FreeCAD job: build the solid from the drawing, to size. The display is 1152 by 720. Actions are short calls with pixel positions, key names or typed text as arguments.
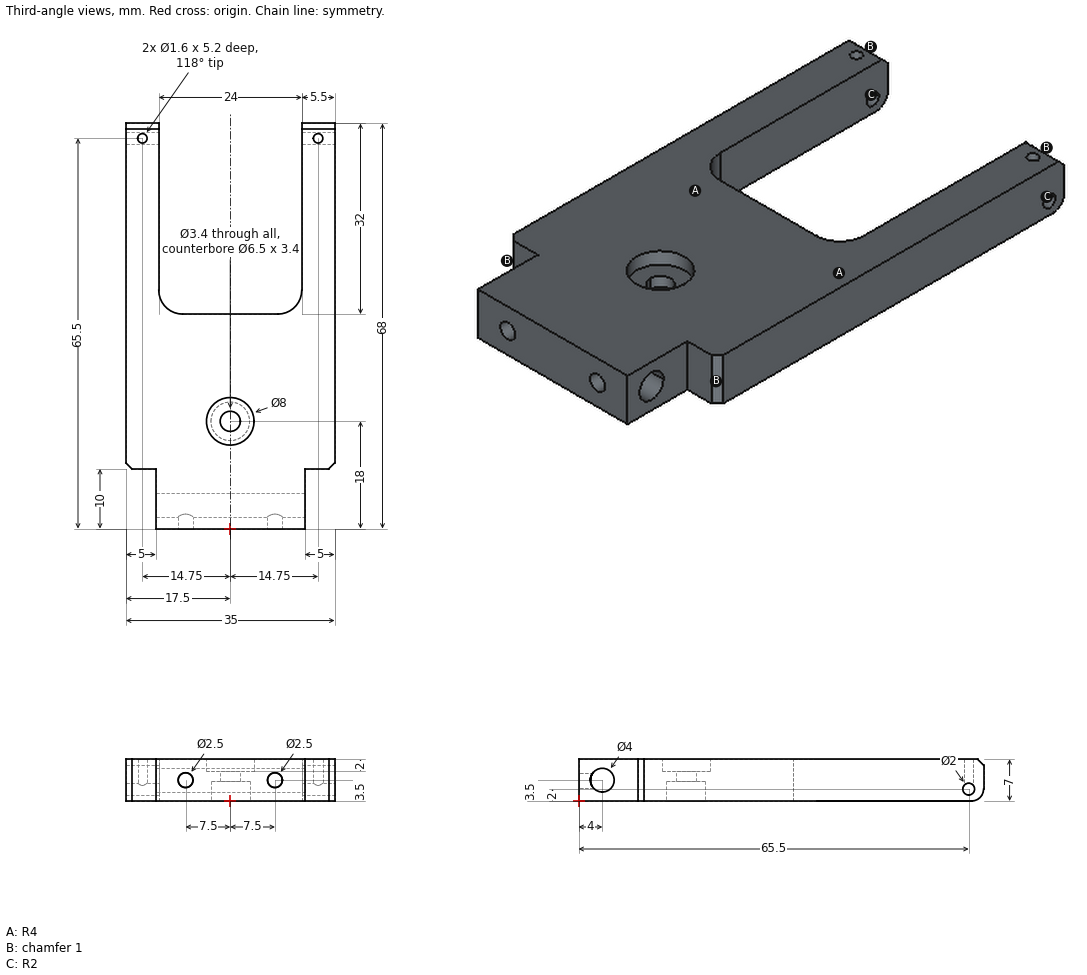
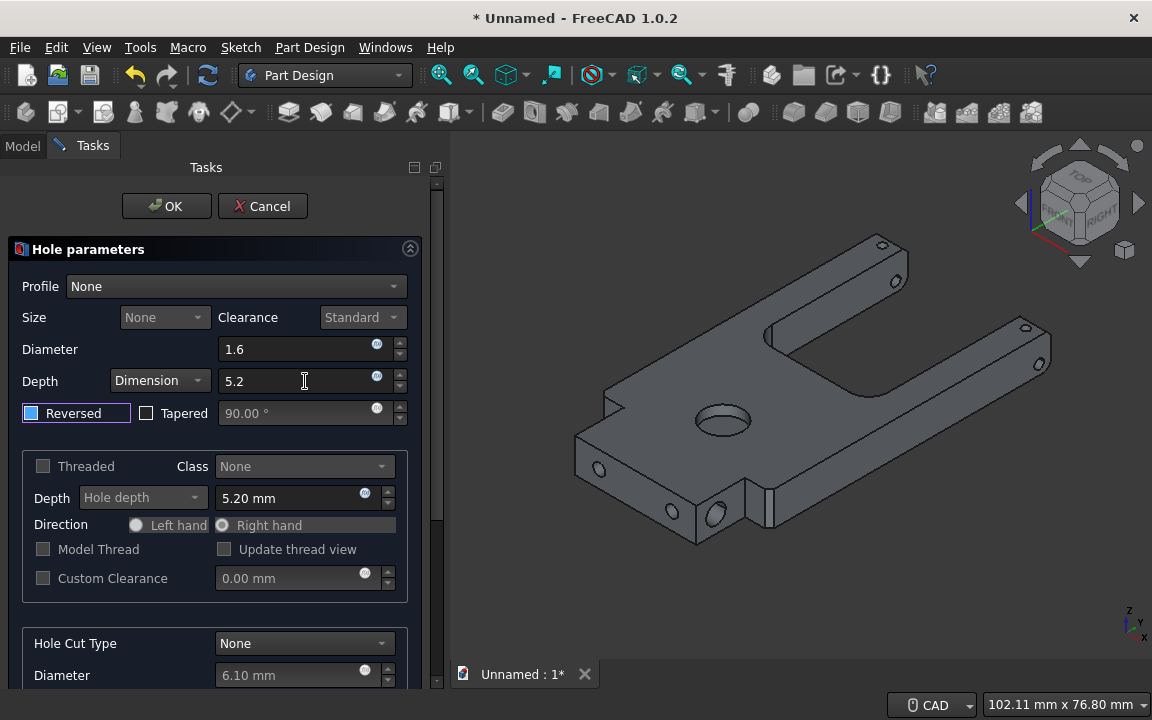
click(167, 206)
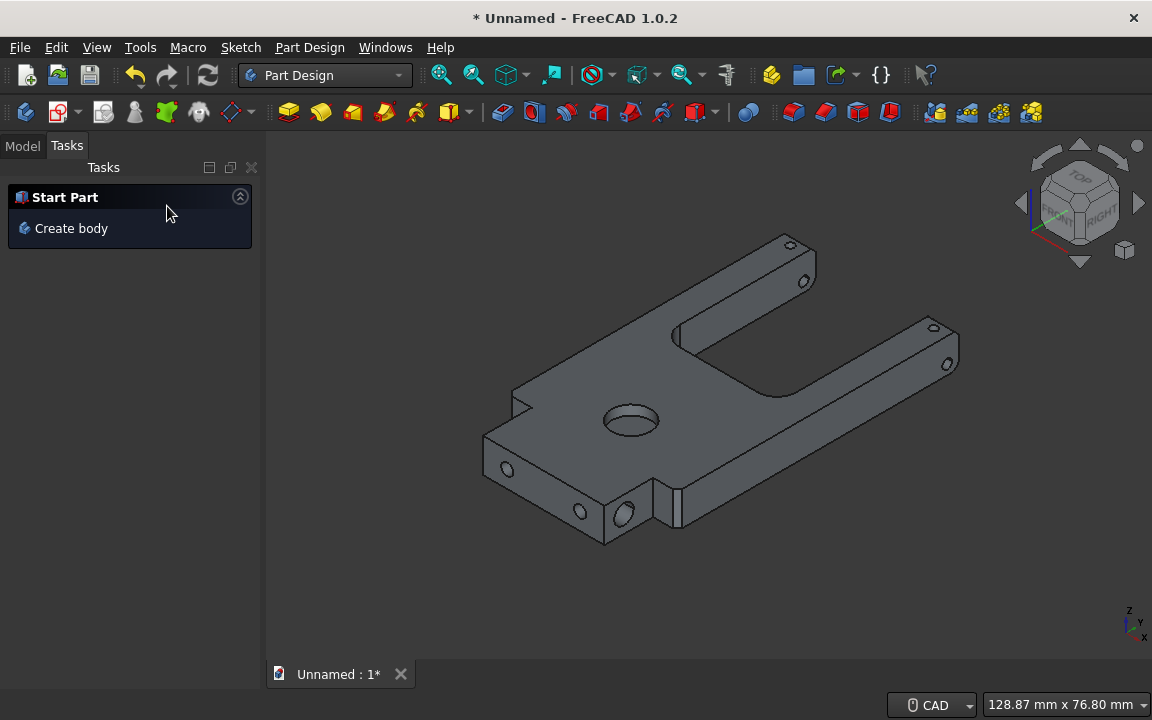
key(5)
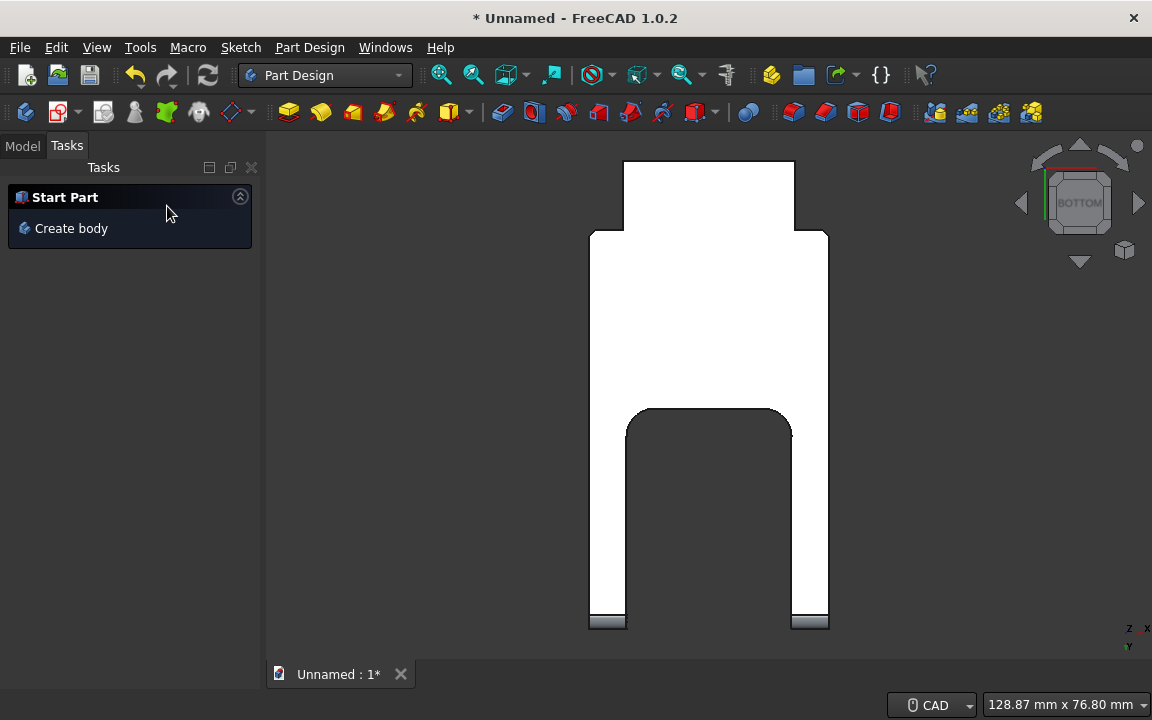
click(709, 257)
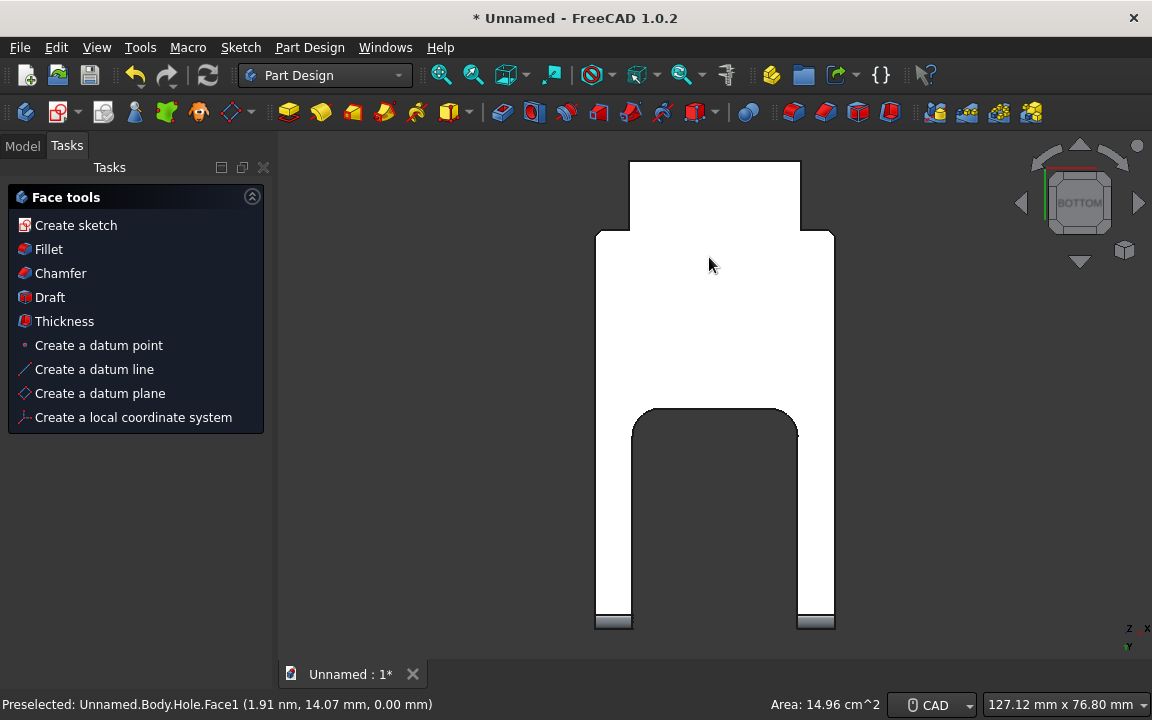
click(58, 112)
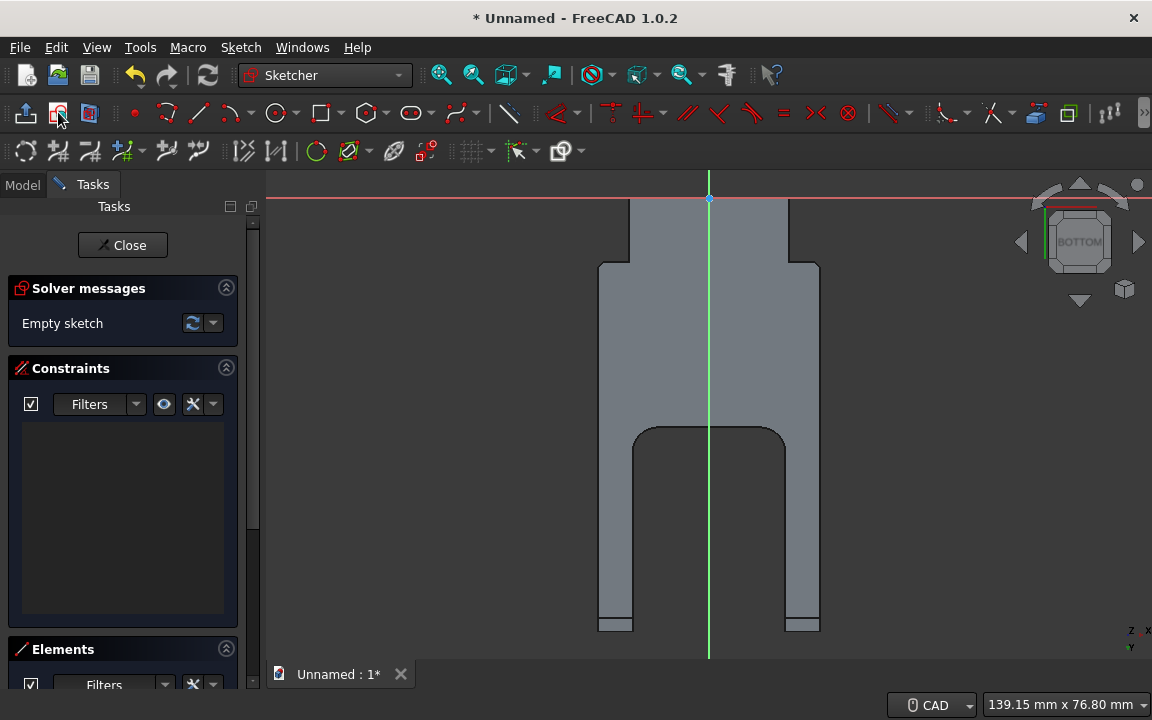
scroll(714, 304, up, 13)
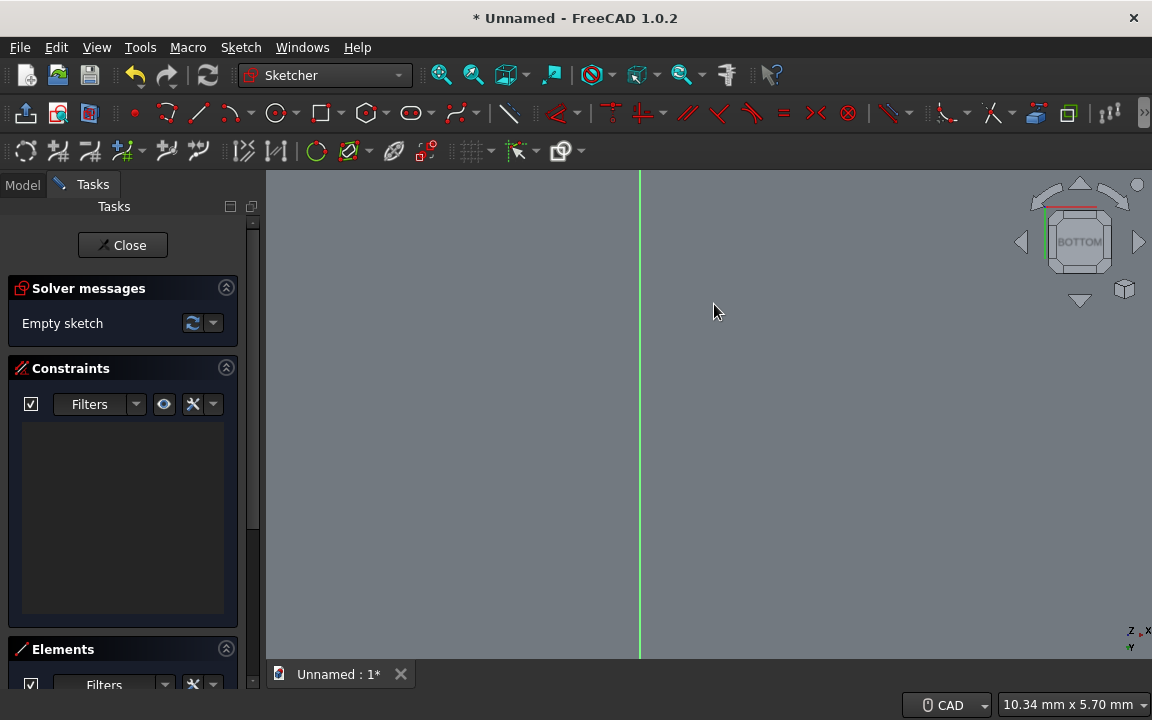
click(276, 114)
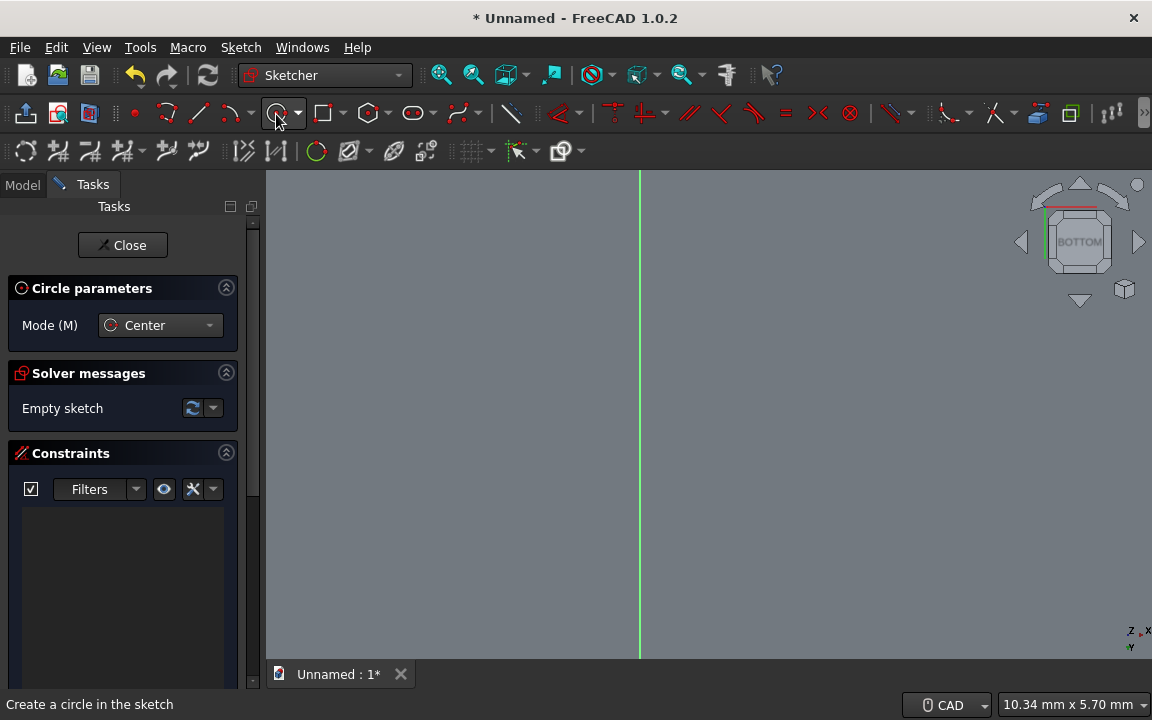
click(640, 417)
move(743, 314)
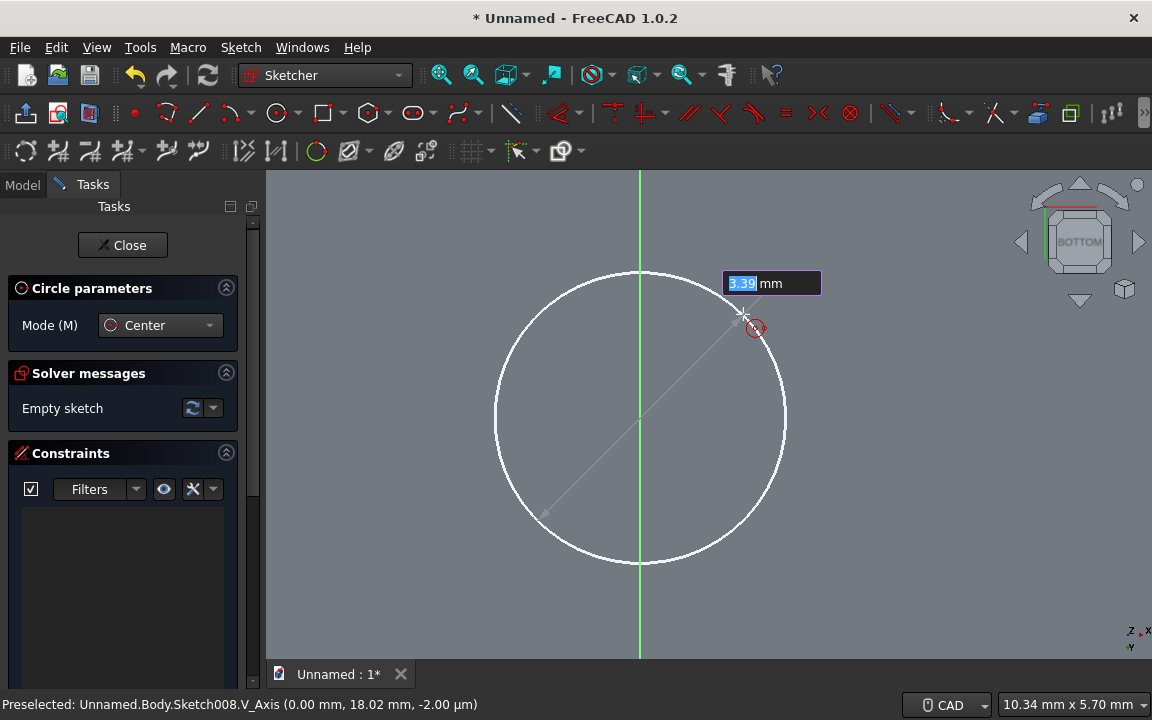
text(3.4)
key(Return)
key(Escape)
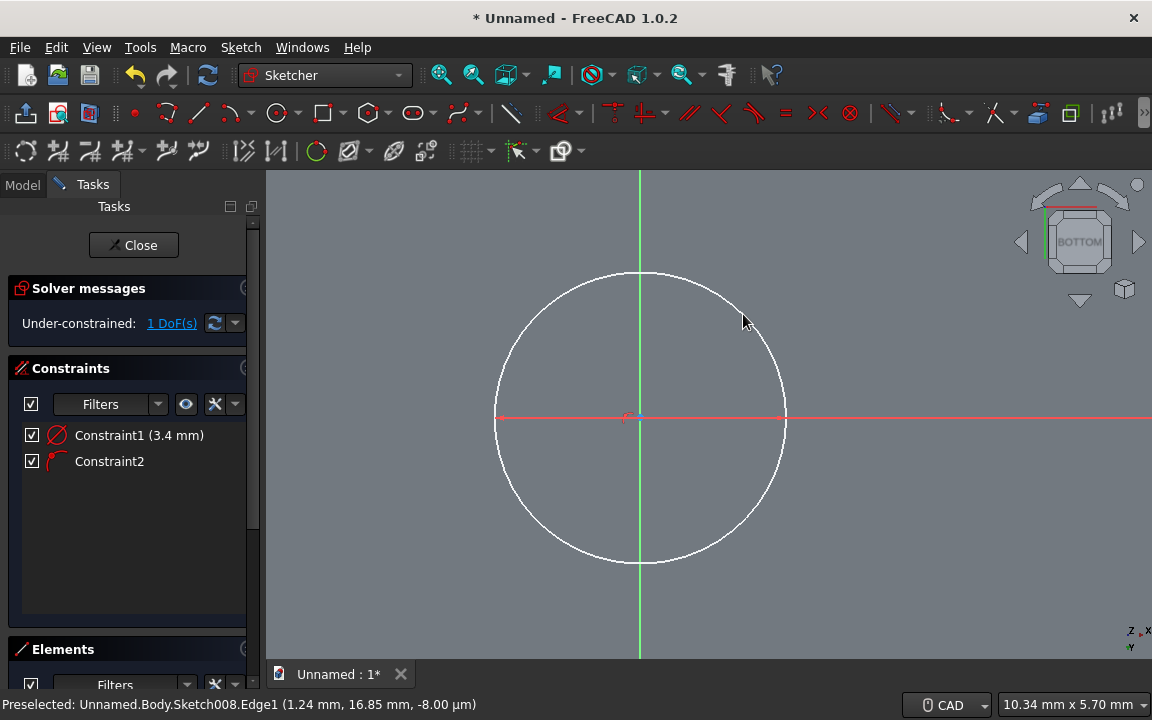
key(d)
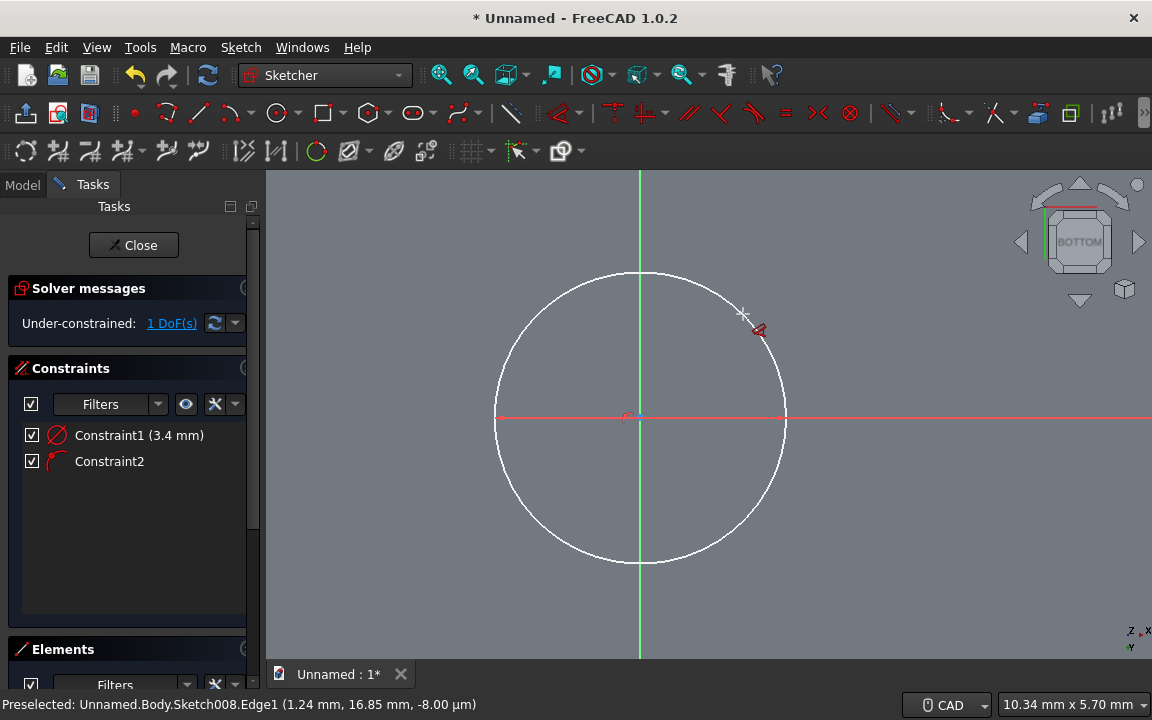
click(640, 418)
click(674, 308)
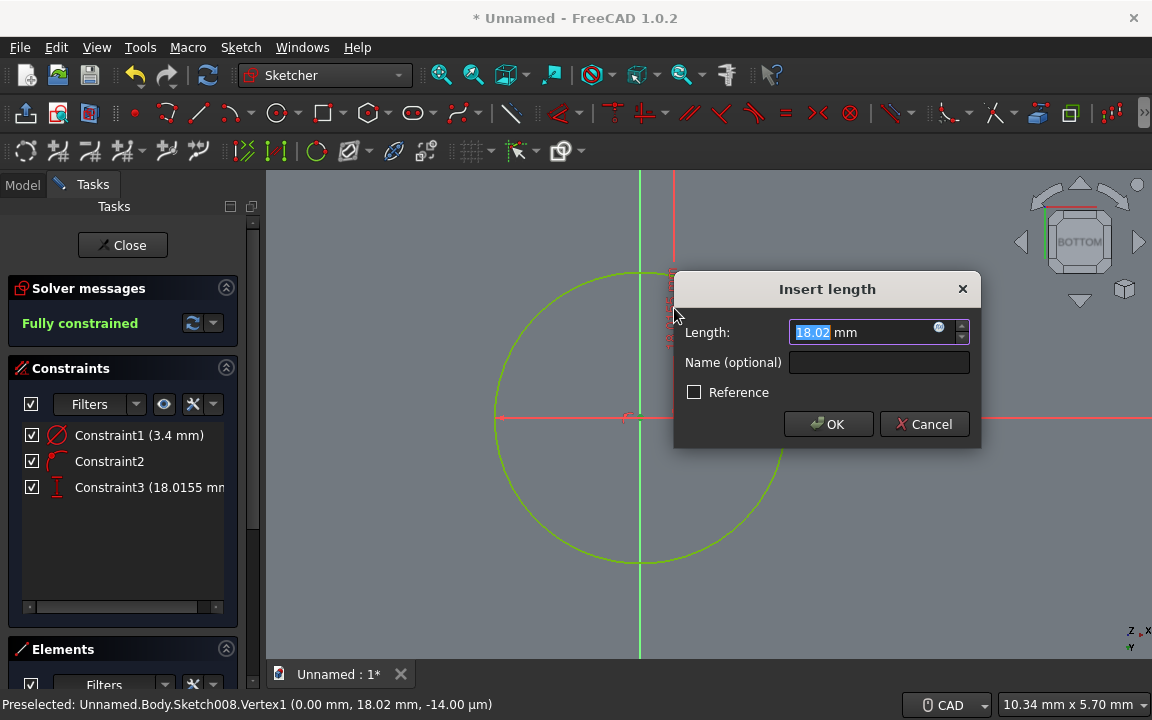
text(18)
key(Return)
key(Escape)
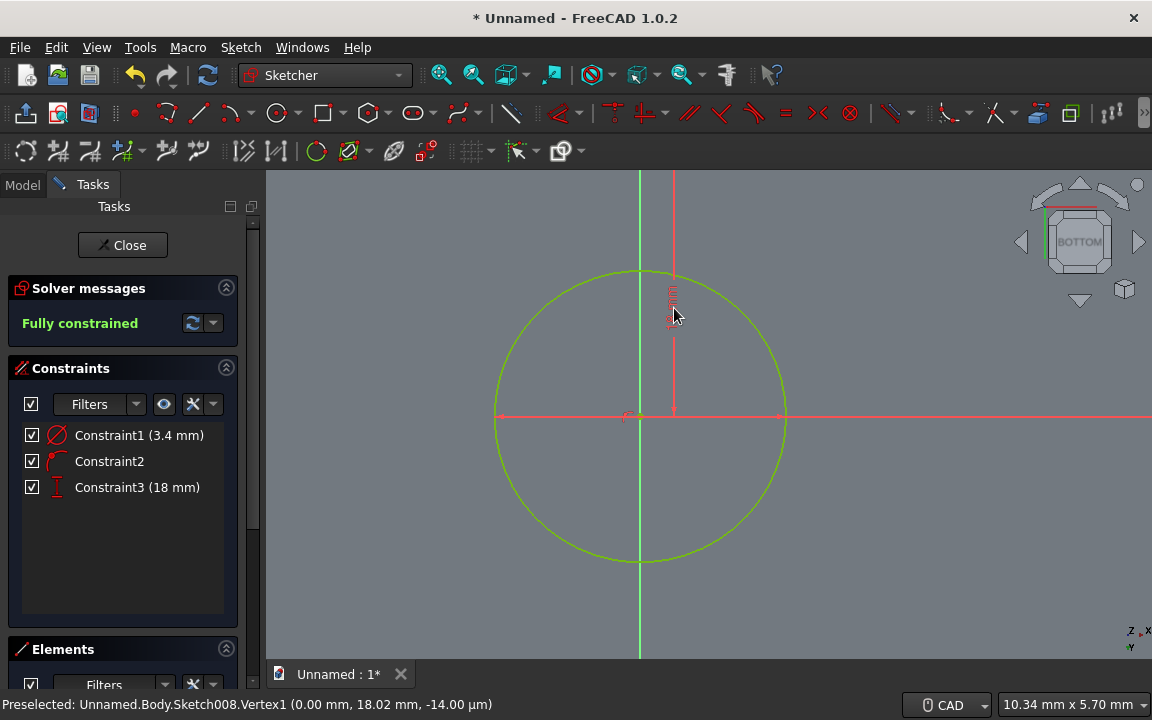
click(123, 245)